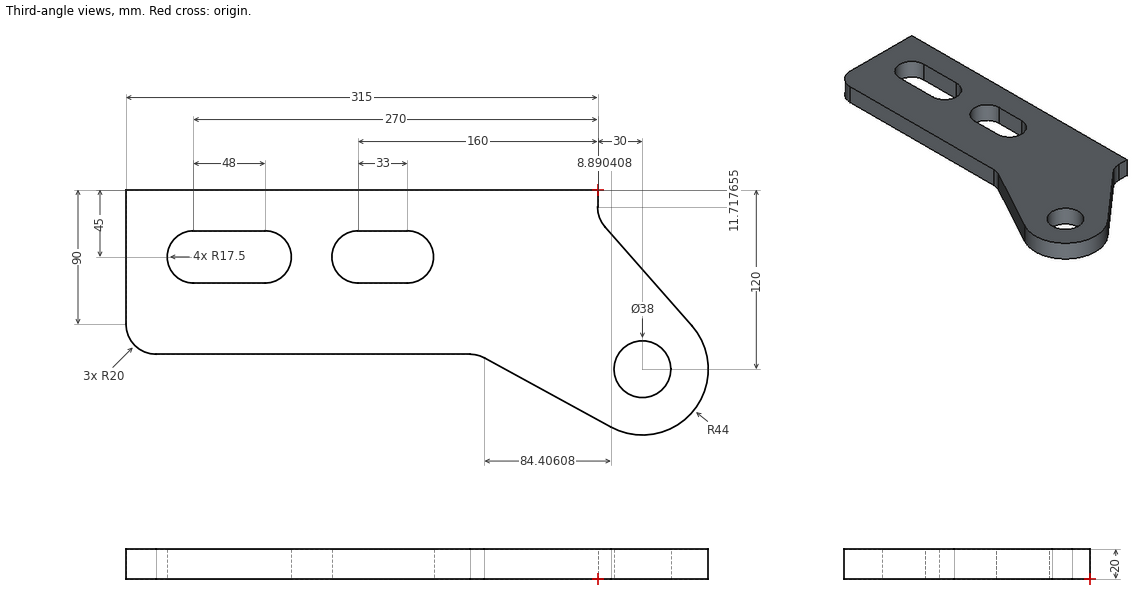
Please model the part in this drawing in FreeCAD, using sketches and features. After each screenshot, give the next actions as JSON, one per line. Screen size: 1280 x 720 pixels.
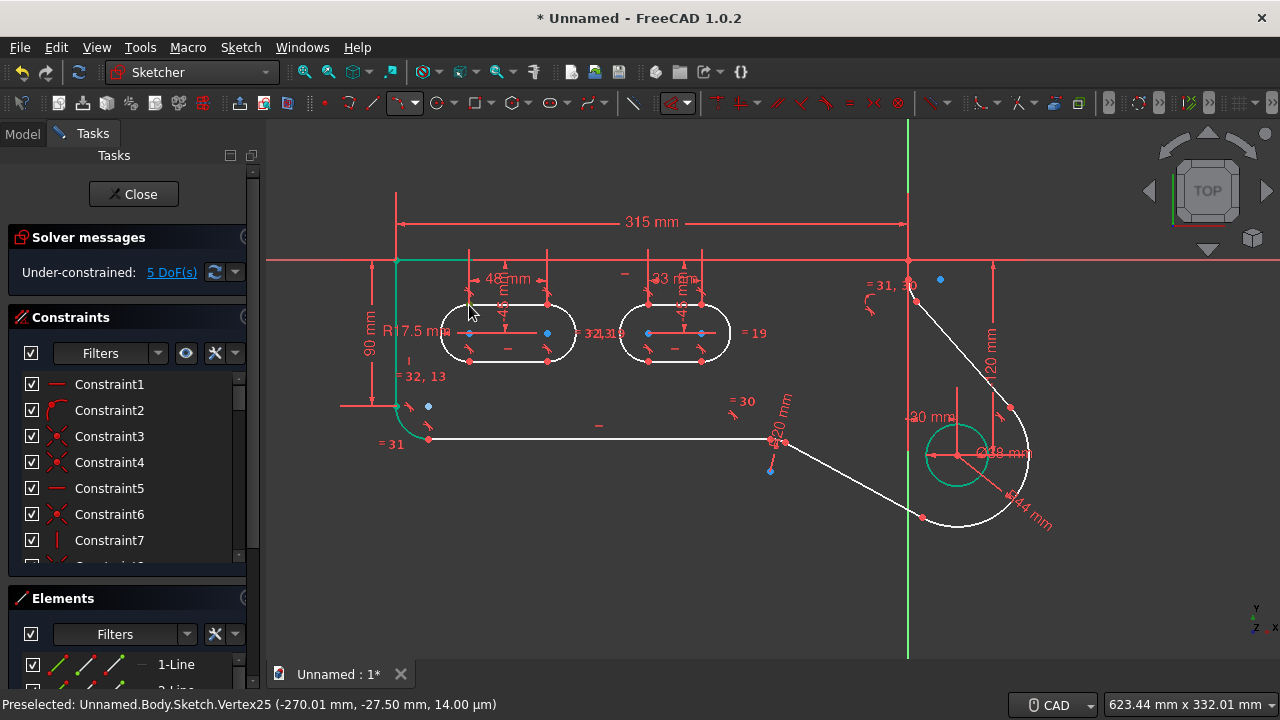
{"action": "left_click", "coordinate": [690, 104]}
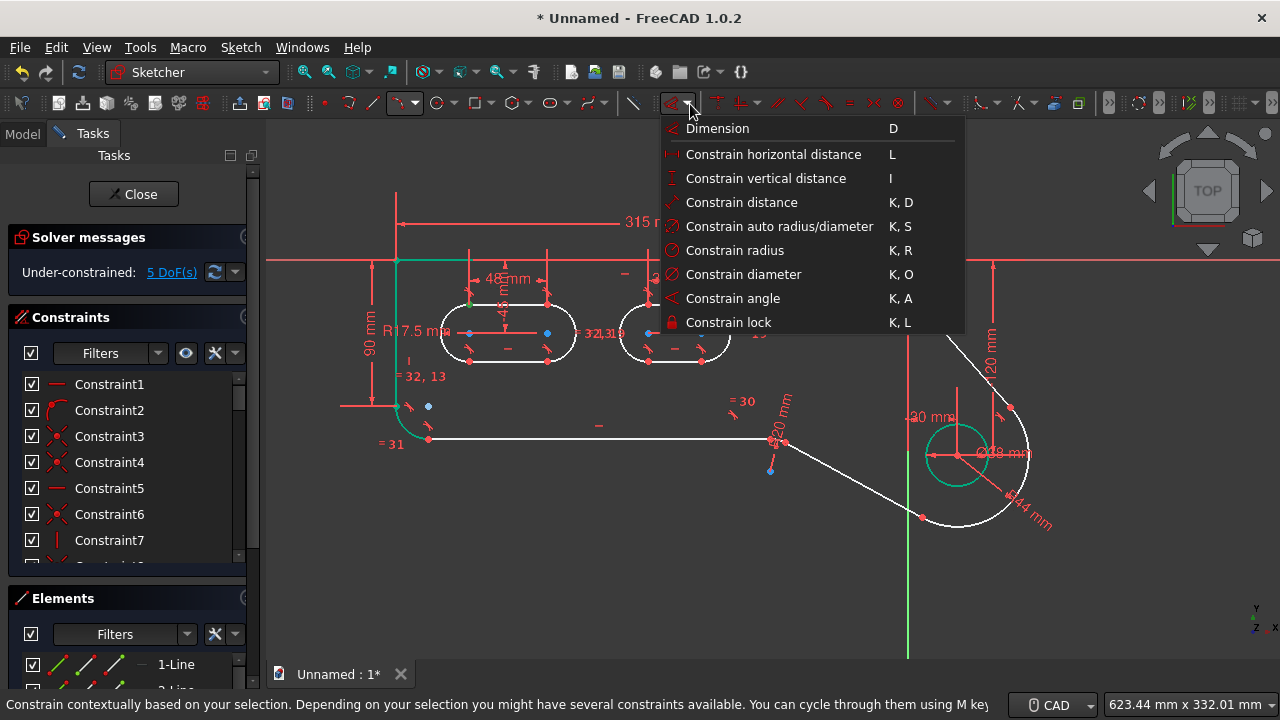
{"action": "left_click", "coordinate": [813, 154]}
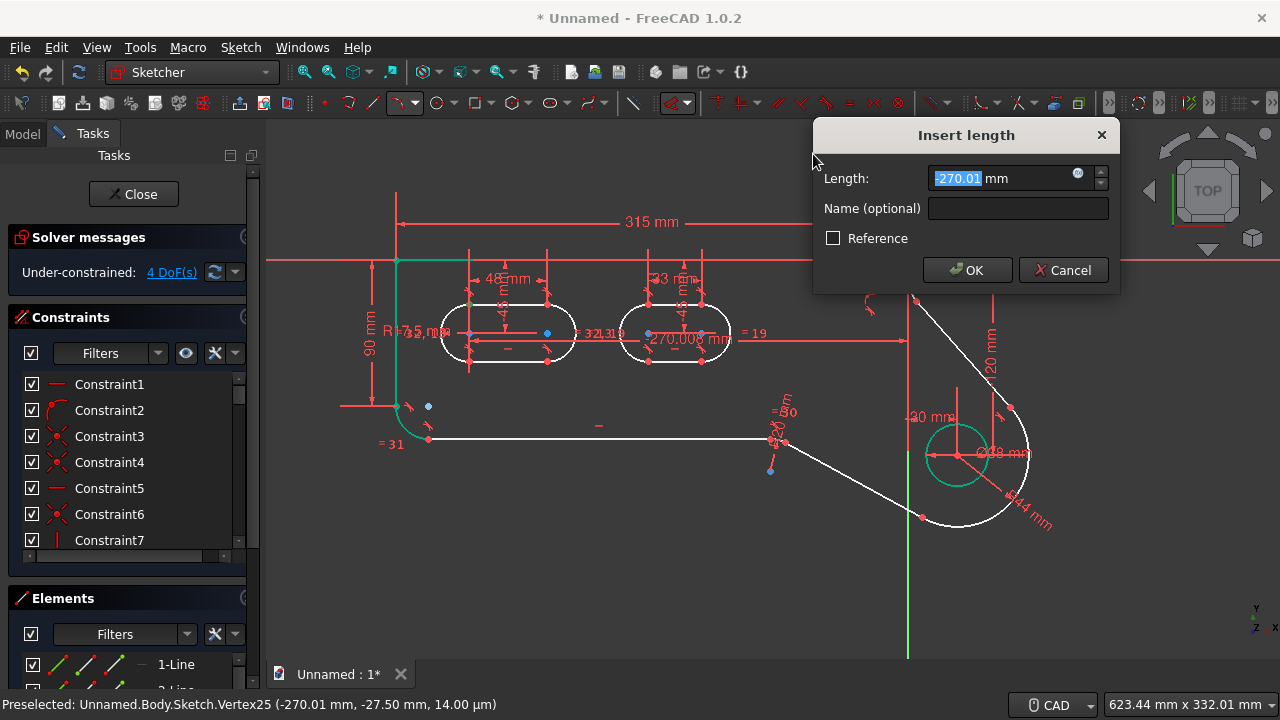
{"action": "type", "text": "-270"}
{"action": "key", "text": "Return"}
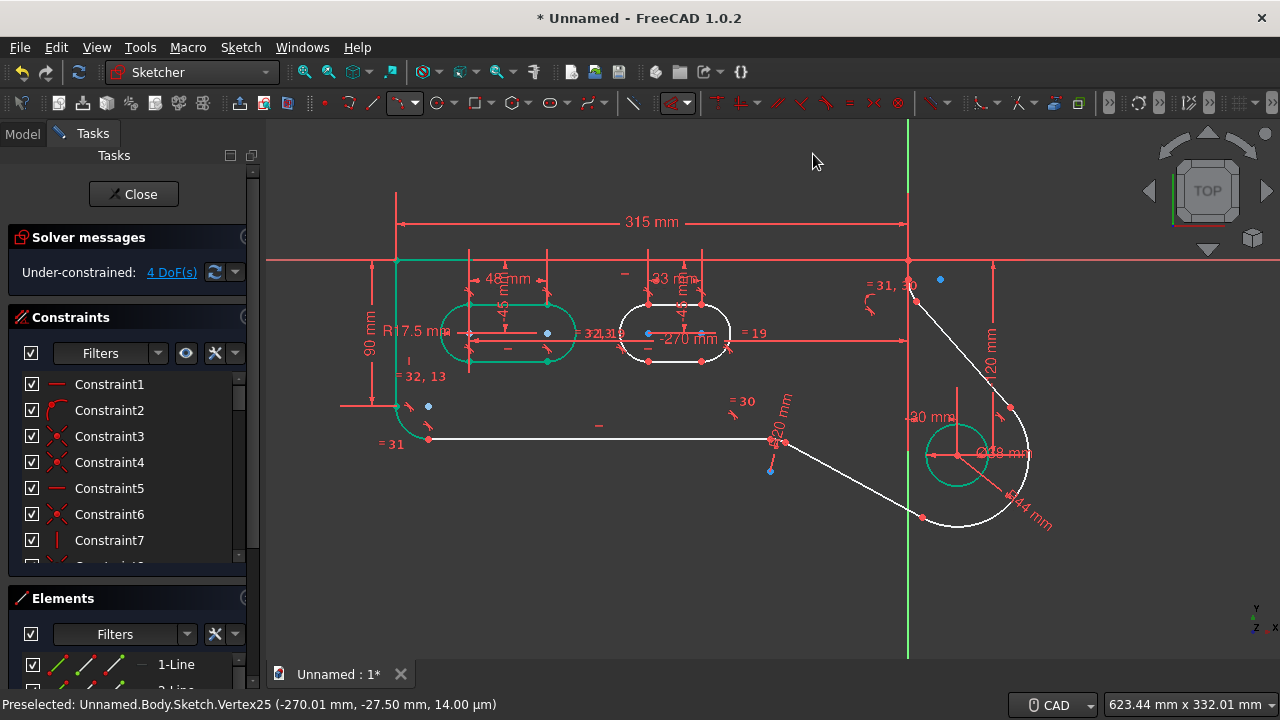
{"action": "left_click", "coordinate": [648, 305]}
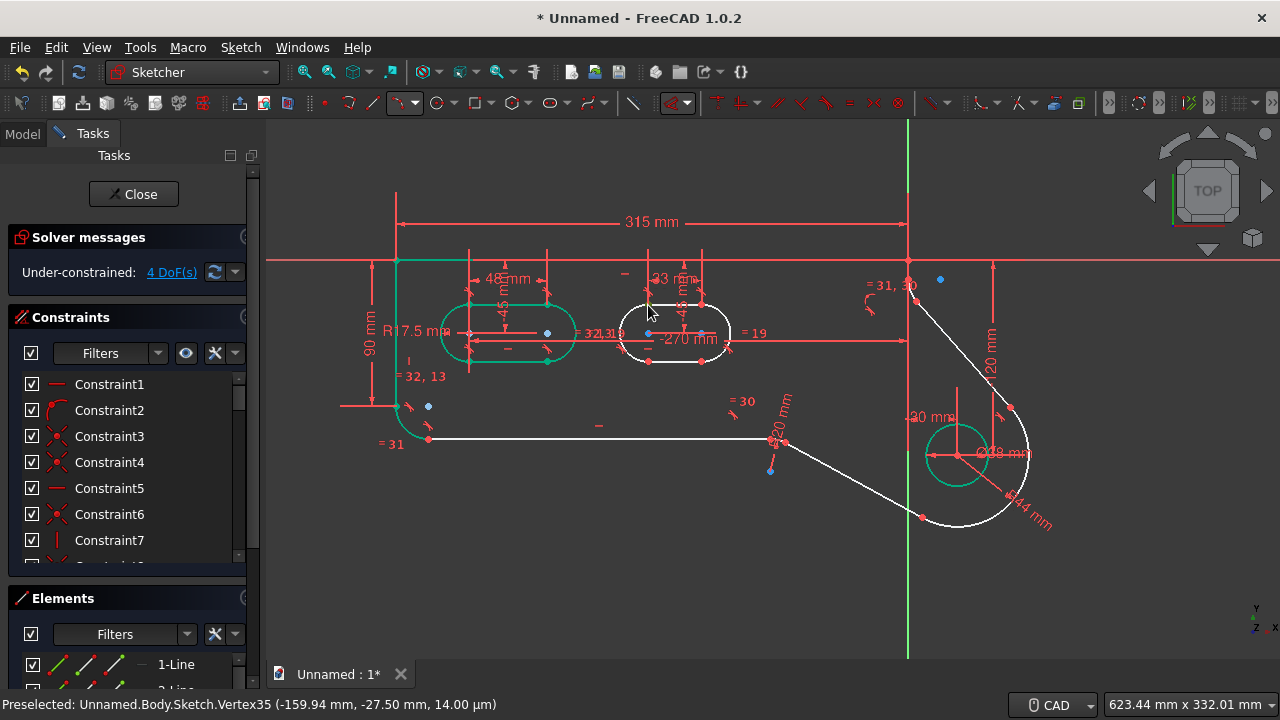
{"action": "left_click", "coordinate": [690, 104]}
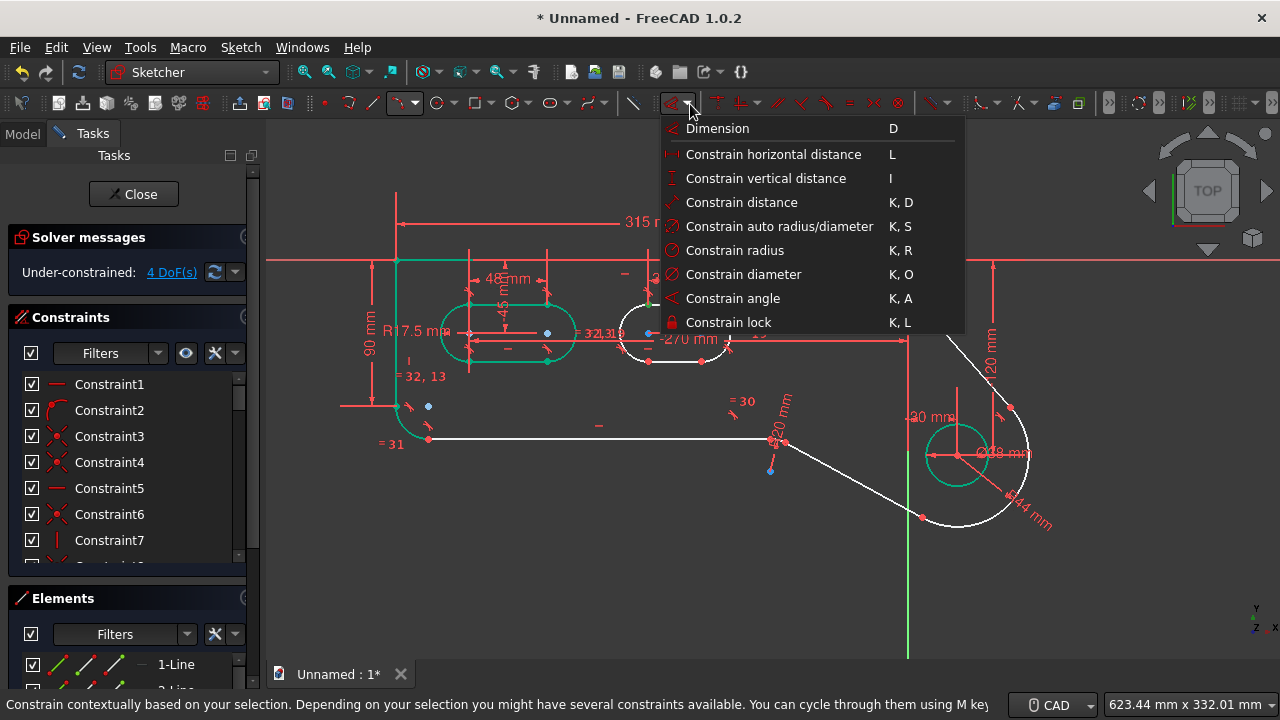
{"action": "left_click", "coordinate": [813, 154]}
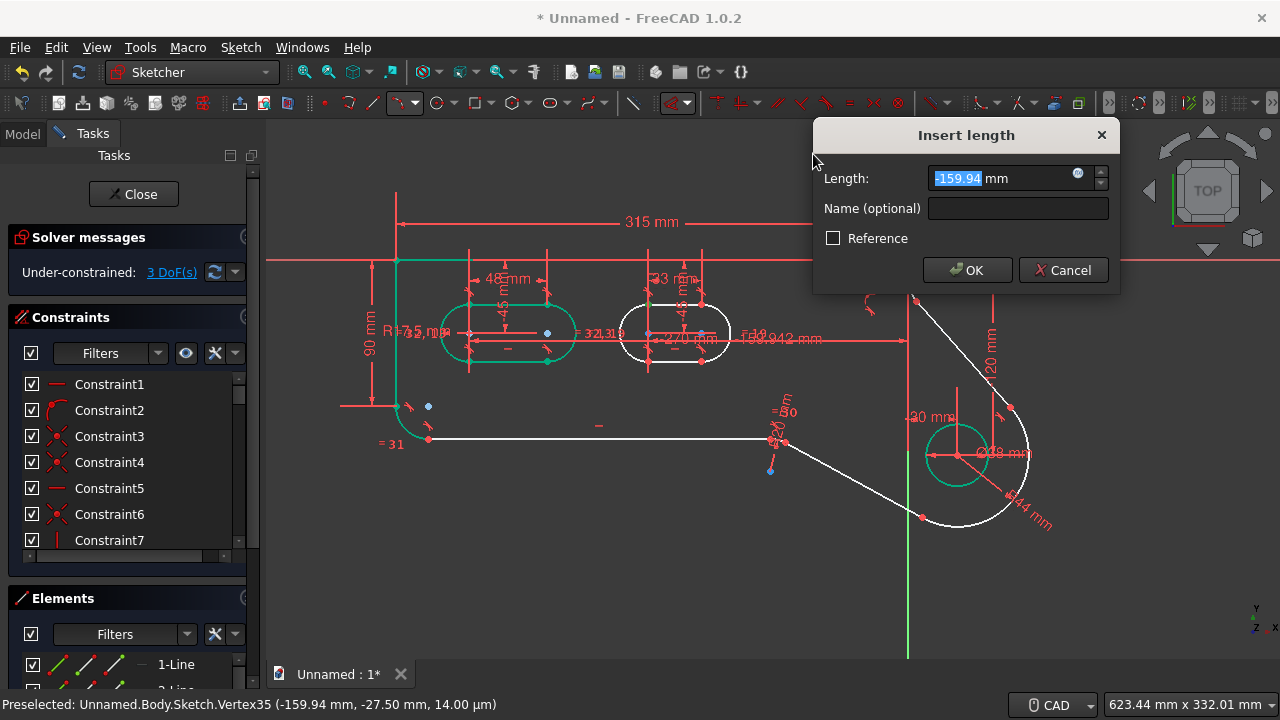
{"action": "type", "text": "-160"}
{"action": "key", "text": "Return"}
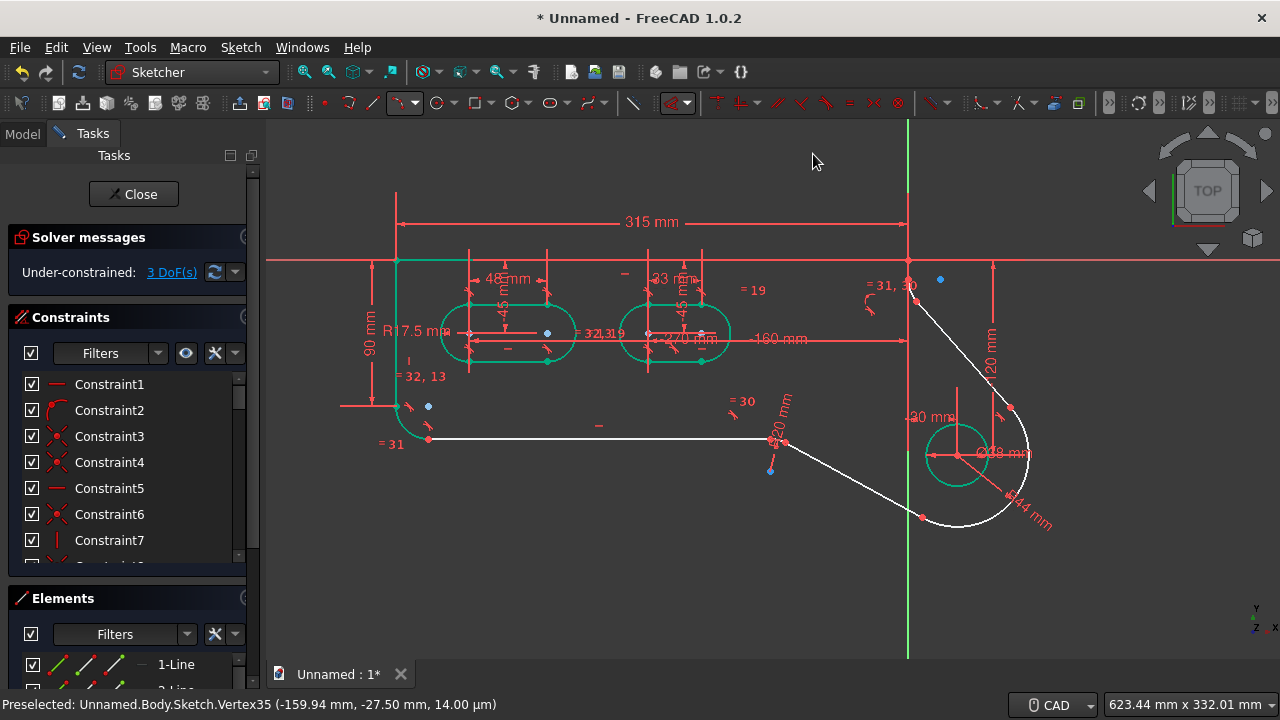
{"action": "scroll", "coordinate": [908, 270], "scroll_direction": "up", "scroll_amount": 4}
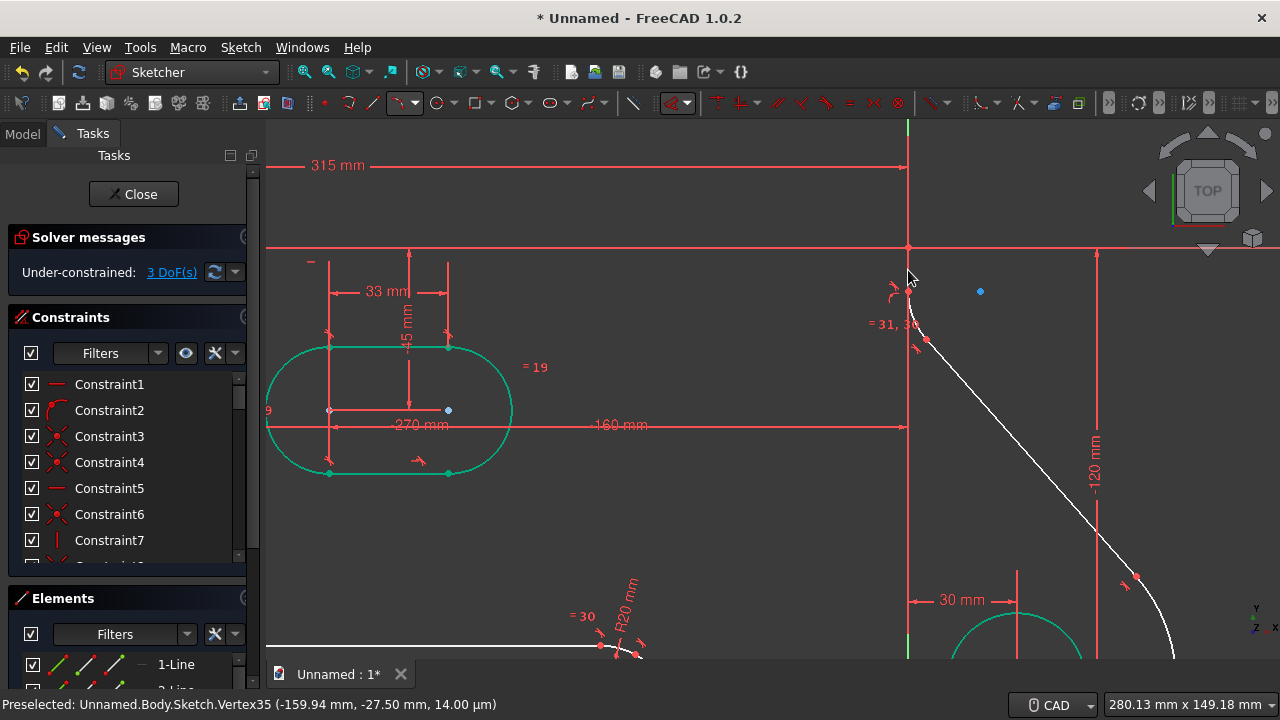
{"action": "left_click", "coordinate": [908, 269]}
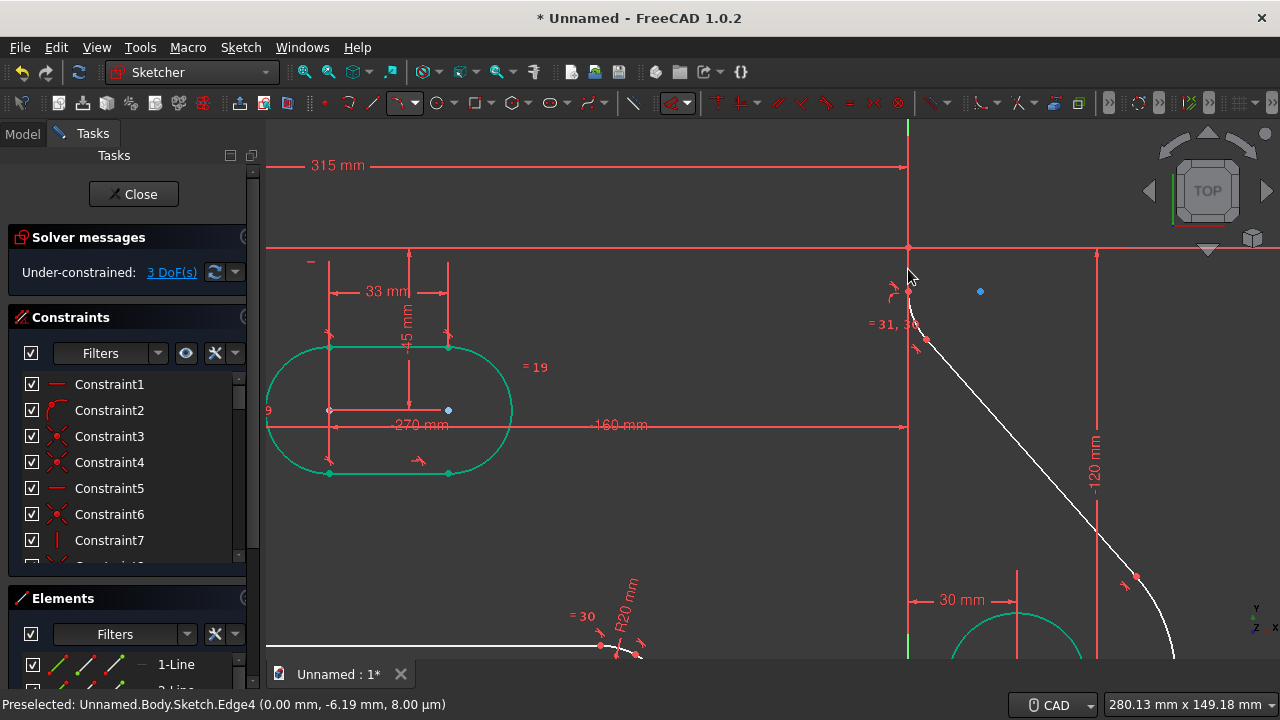
{"action": "left_click", "coordinate": [690, 104]}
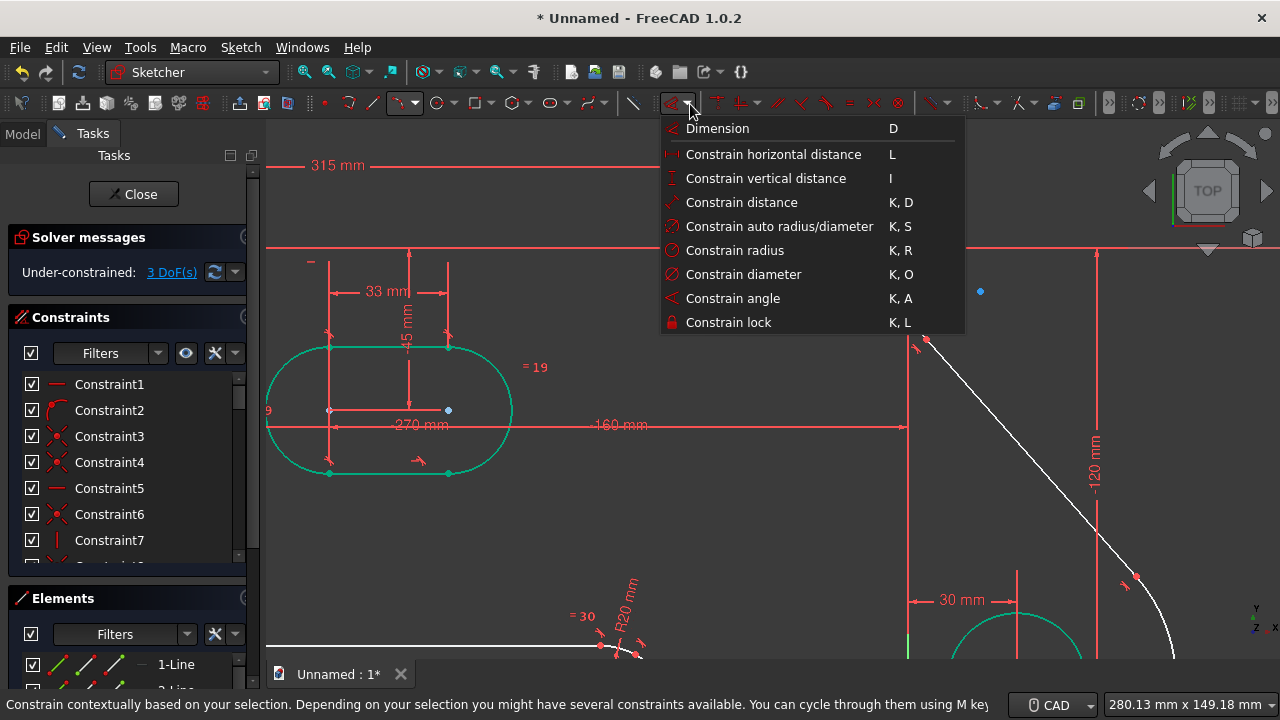
{"action": "left_click", "coordinate": [813, 178]}